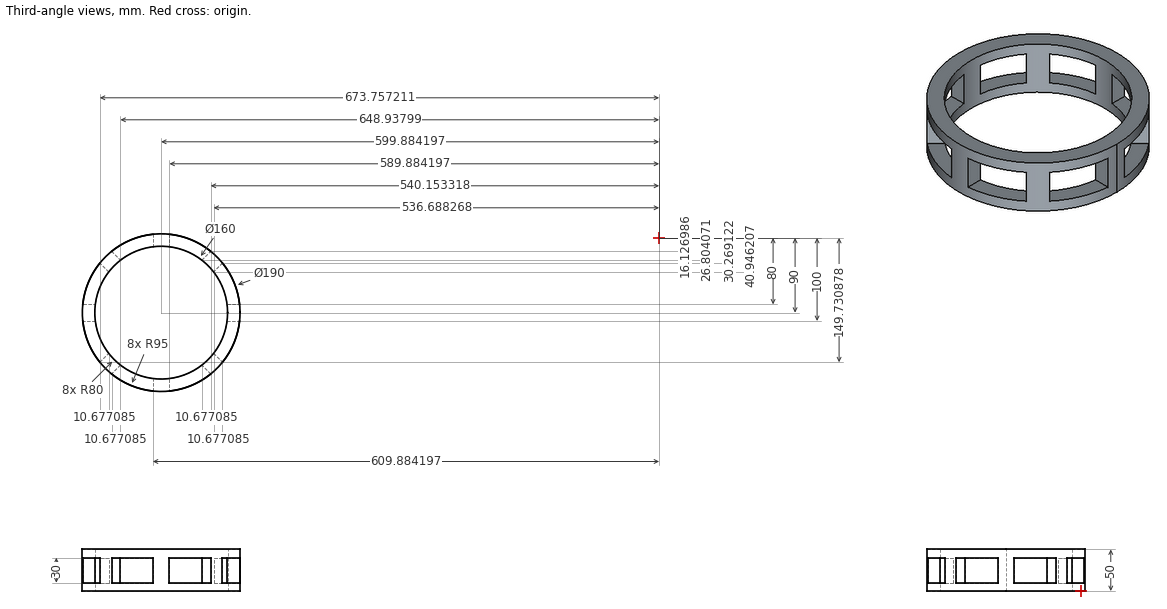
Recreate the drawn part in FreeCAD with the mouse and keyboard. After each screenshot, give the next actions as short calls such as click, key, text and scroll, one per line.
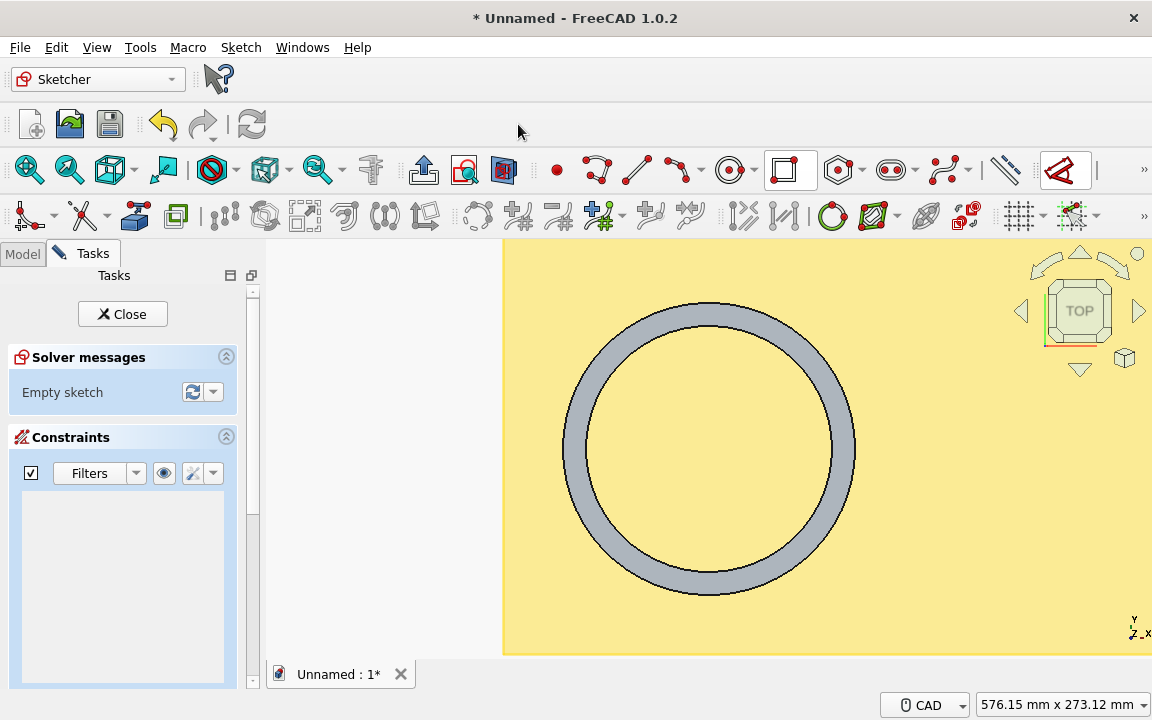
key(q)
key(s)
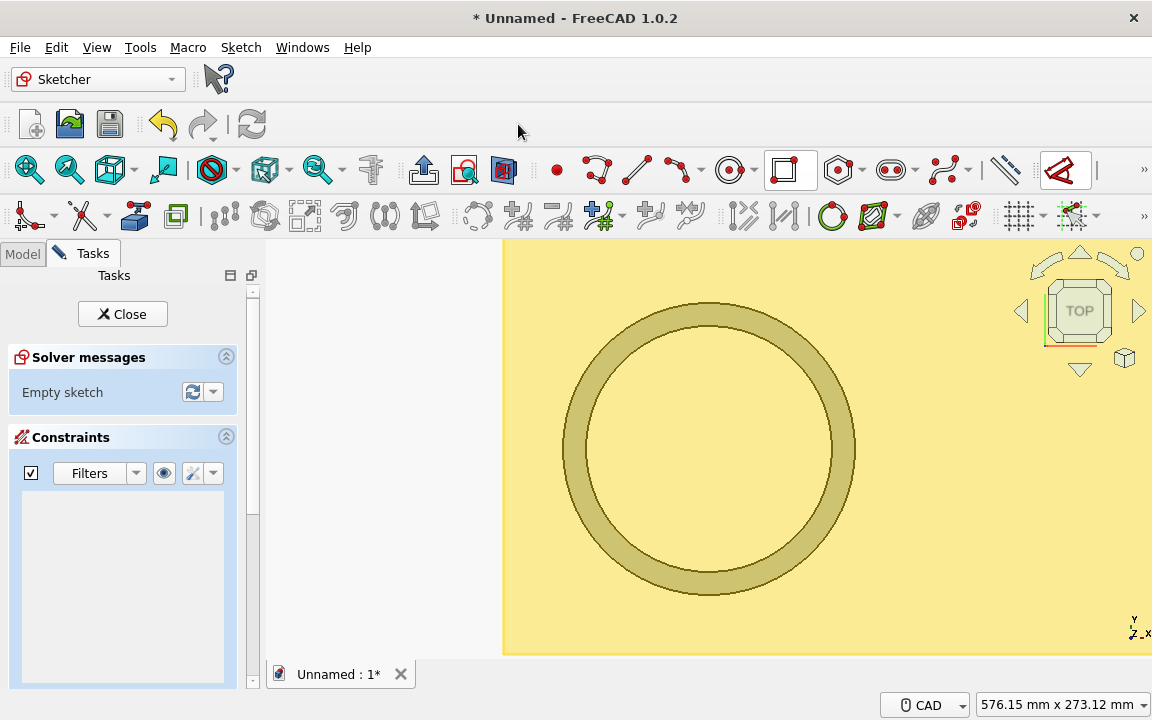
key(g)
key(l)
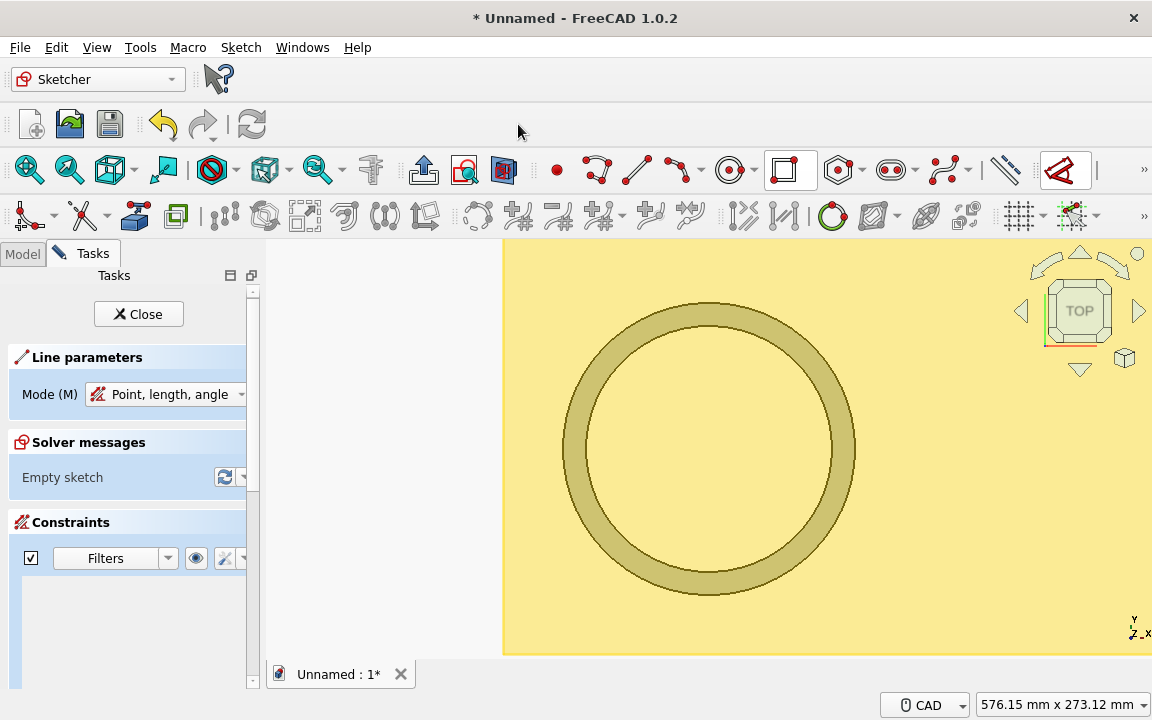
click(595, 541)
click(612, 524)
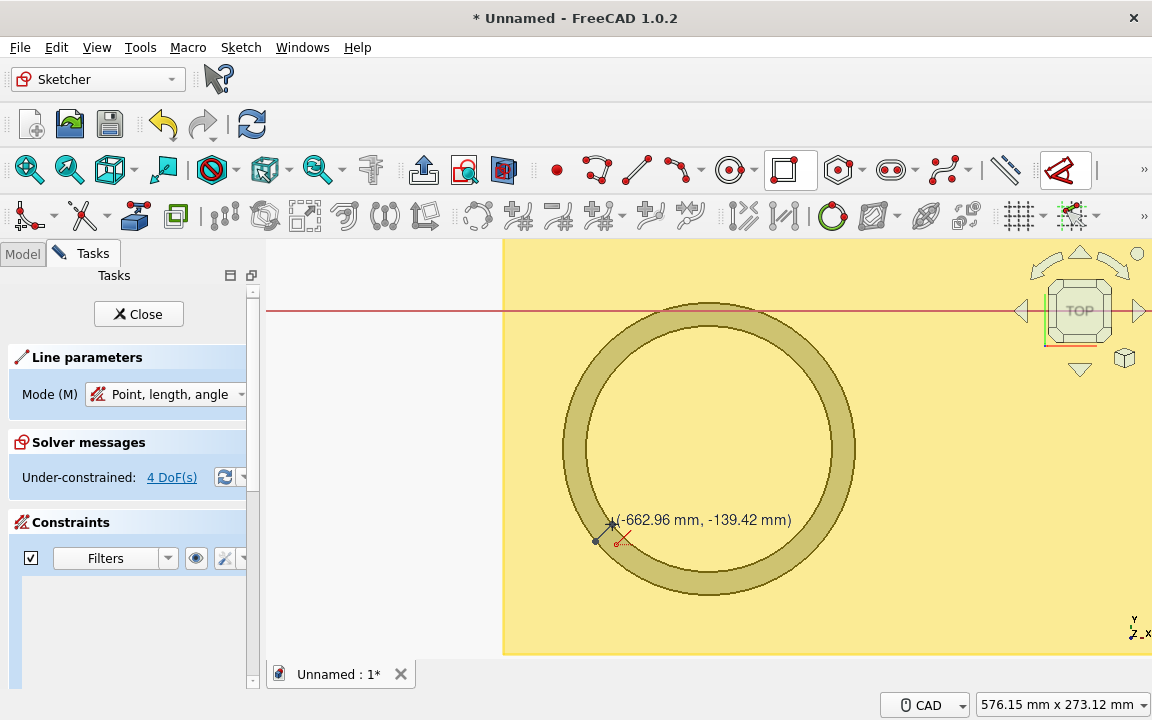
click(634, 546)
click(617, 563)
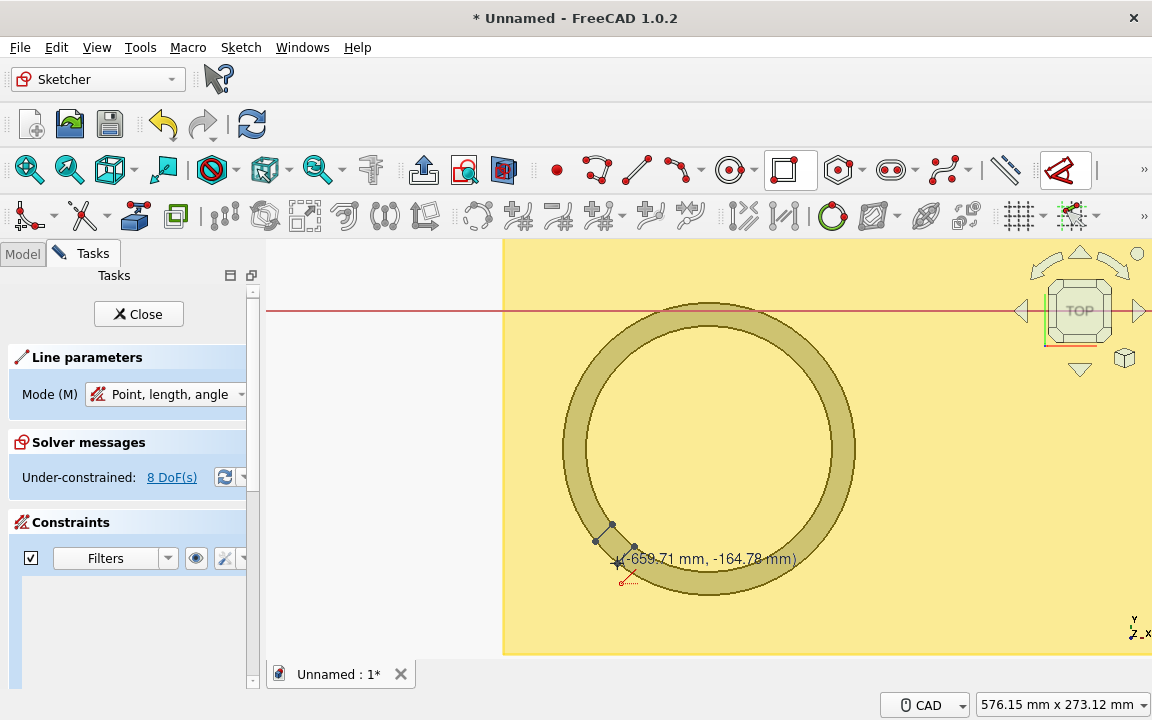
click(694, 594)
click(694, 571)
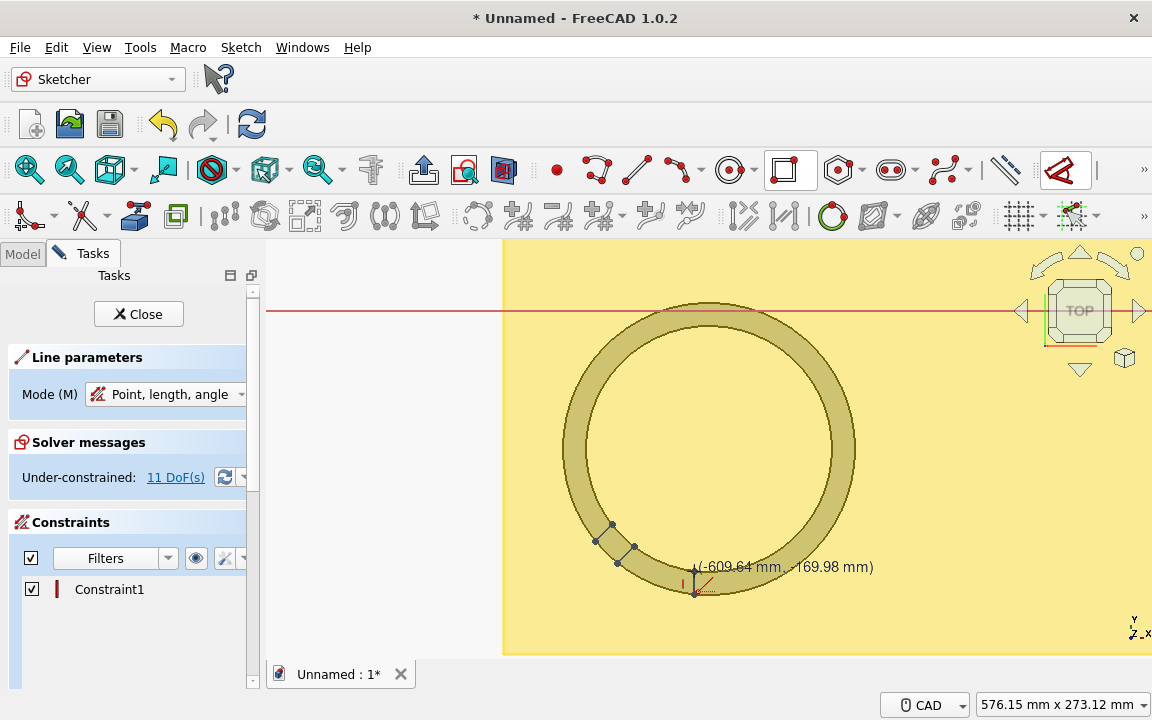
click(724, 571)
click(724, 594)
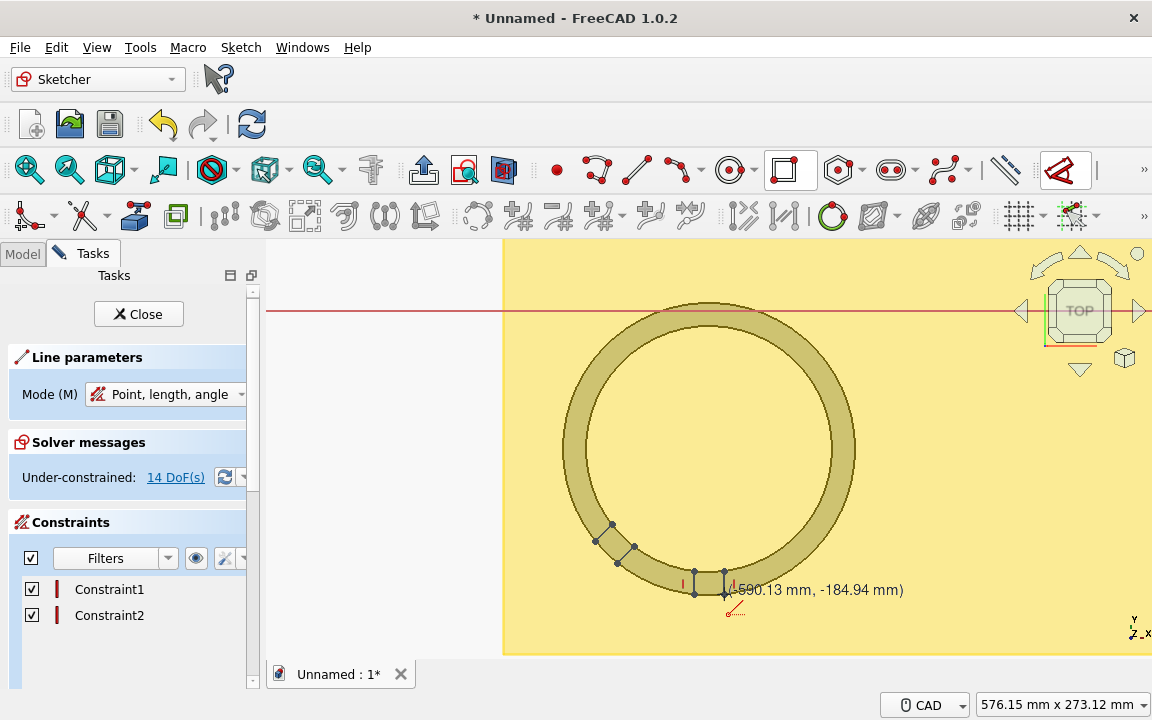
click(801, 563)
click(784, 546)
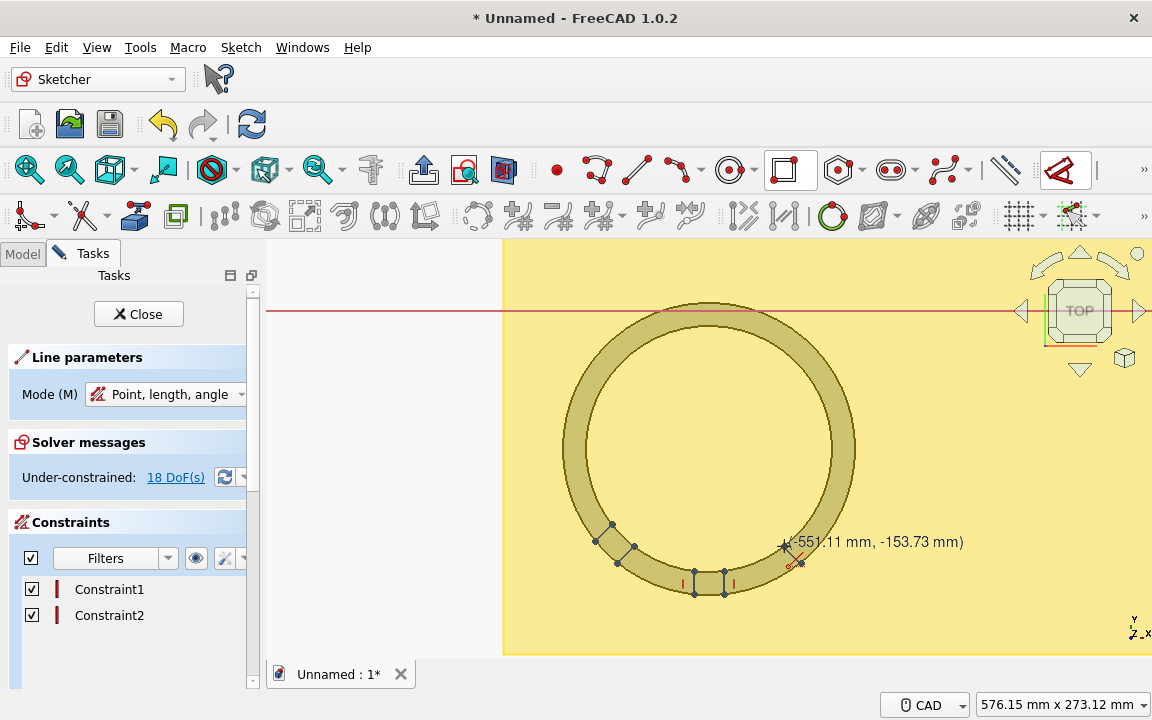
click(806, 524)
click(823, 541)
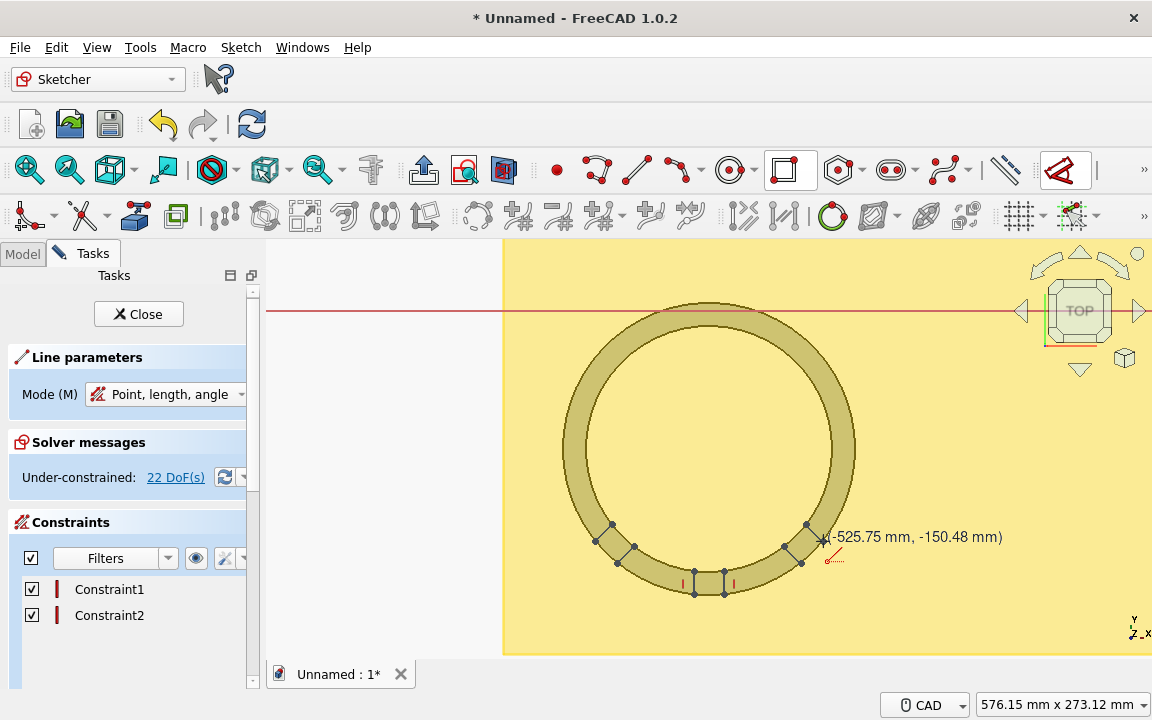
click(854, 464)
click(831, 464)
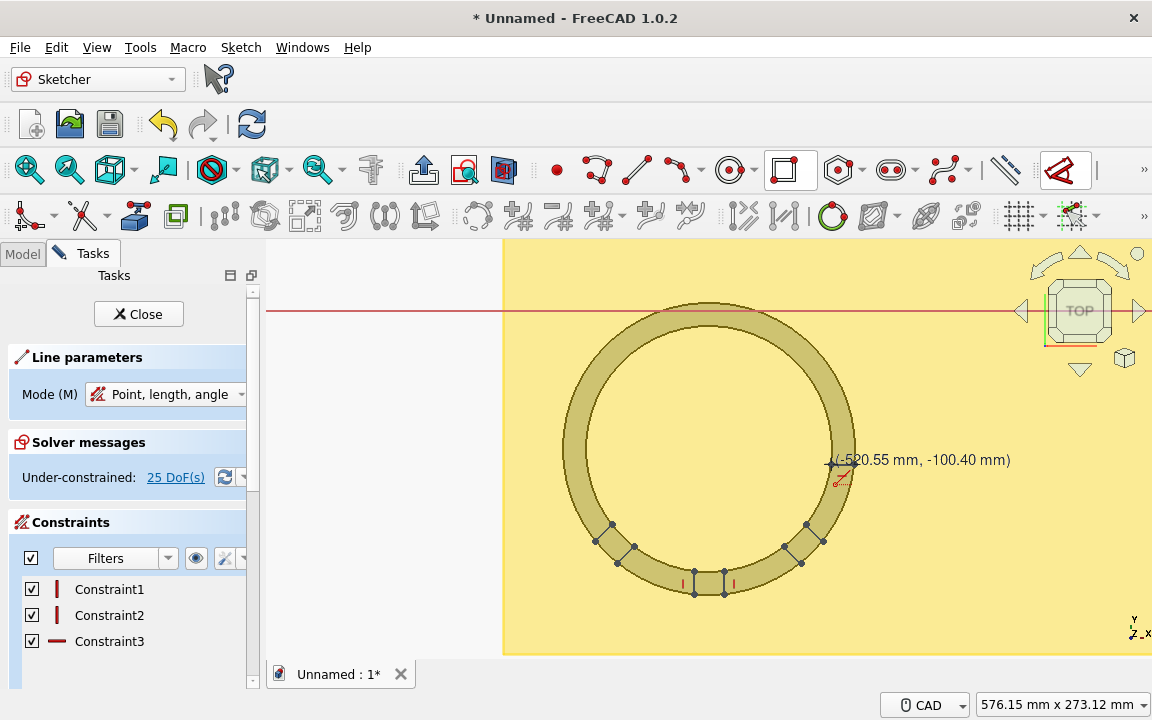
click(831, 434)
click(854, 434)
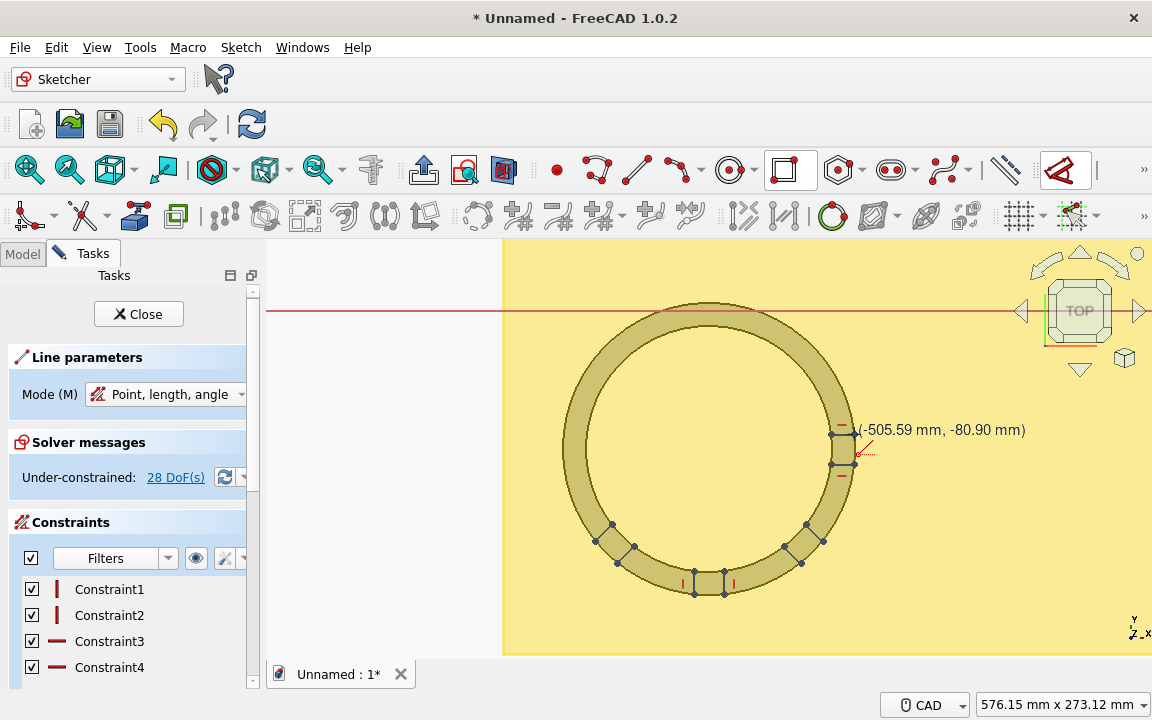
click(823, 357)
click(806, 374)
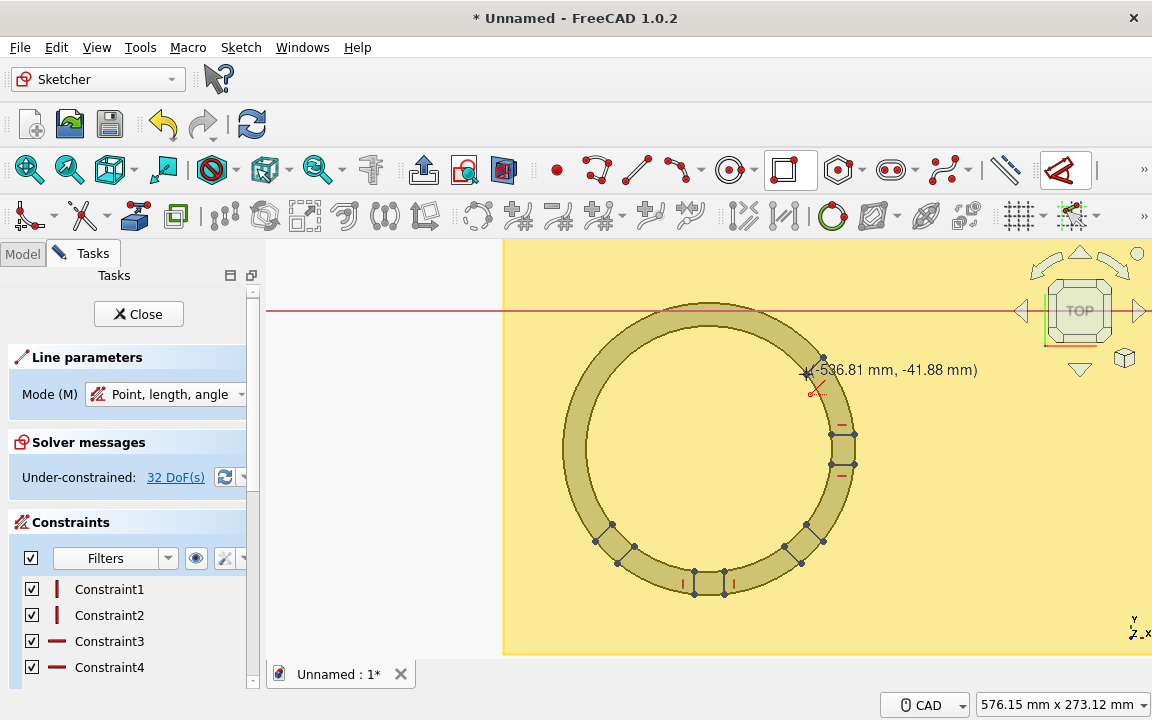
click(784, 352)
click(801, 335)